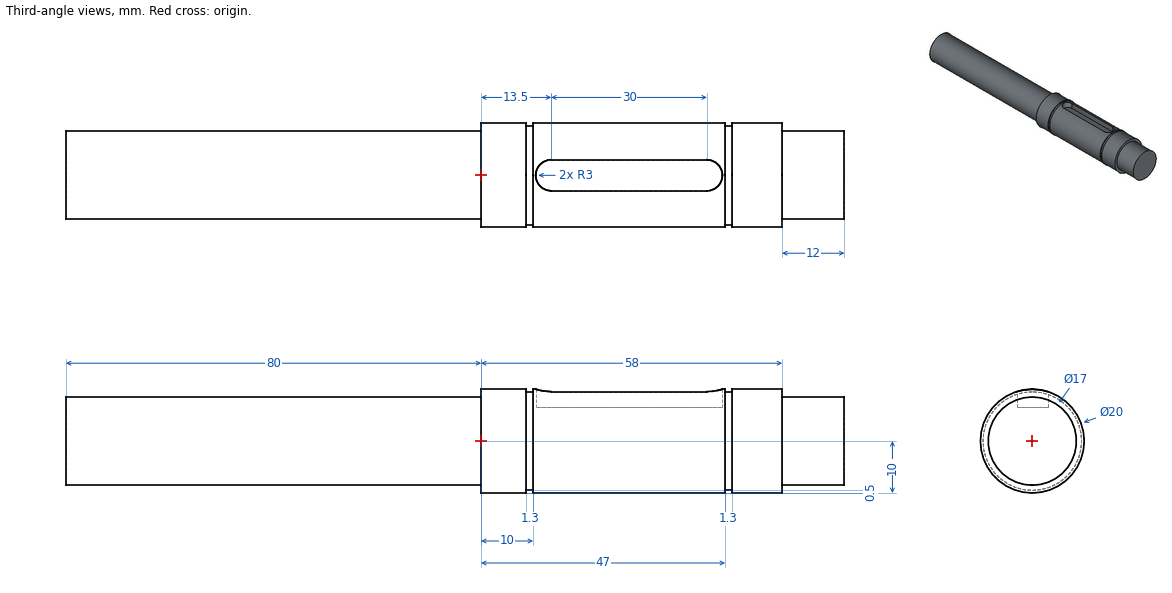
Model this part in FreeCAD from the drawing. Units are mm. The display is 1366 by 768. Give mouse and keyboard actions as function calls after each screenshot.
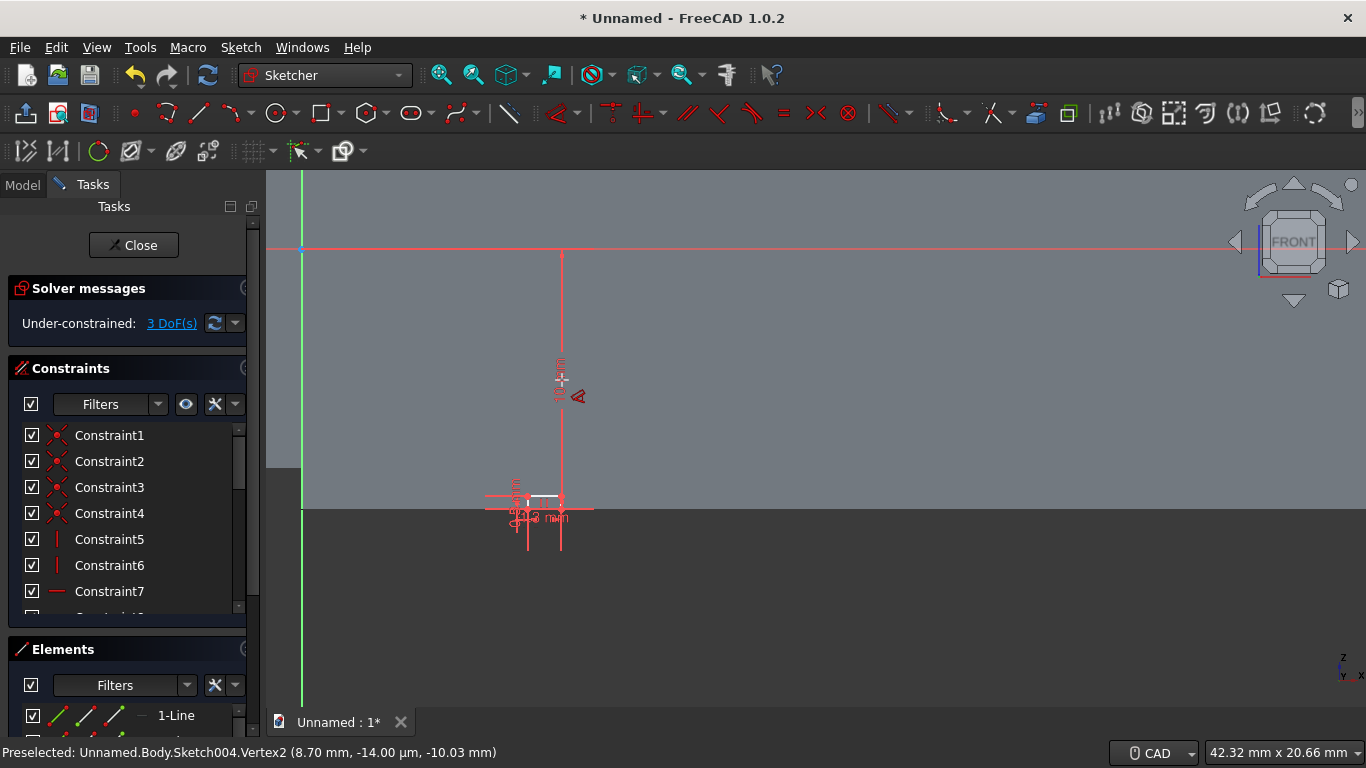
click(561, 509)
click(431, 215)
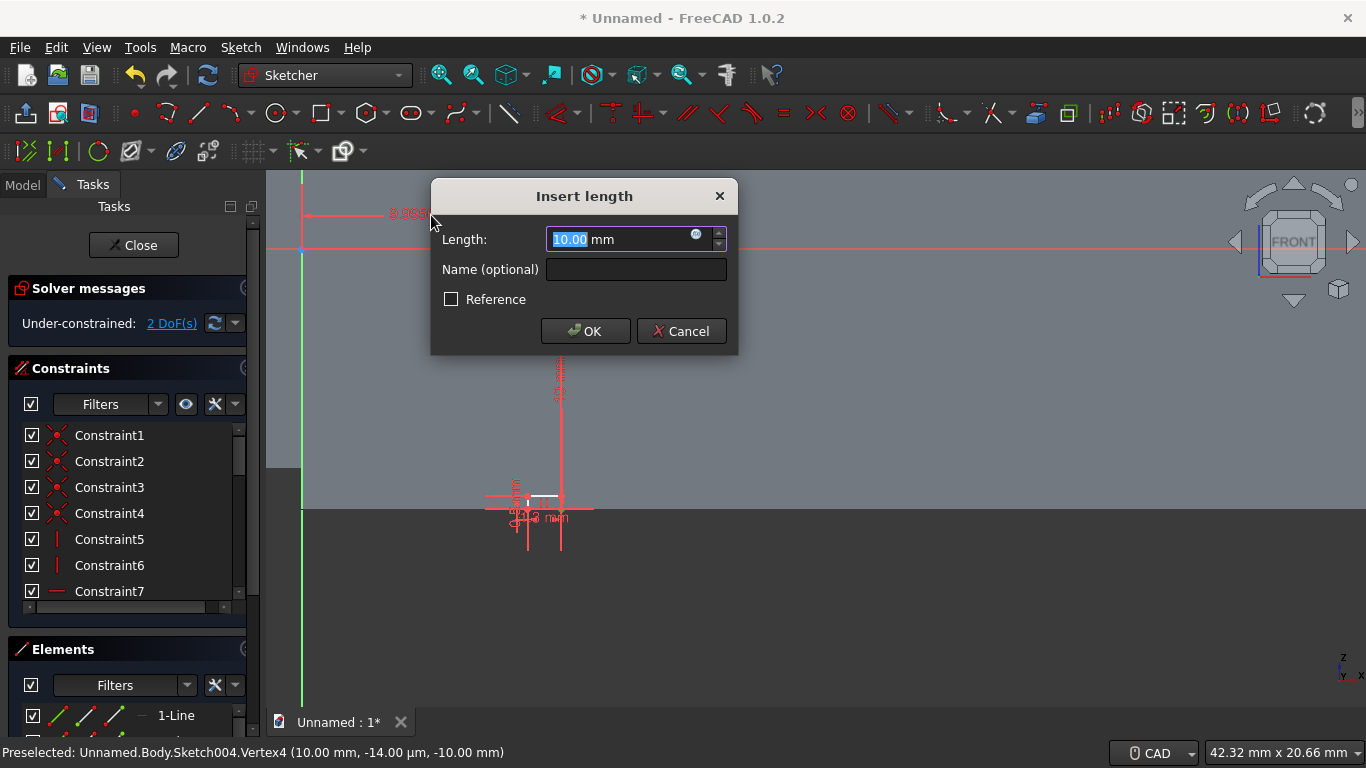
text(10)
key(Return)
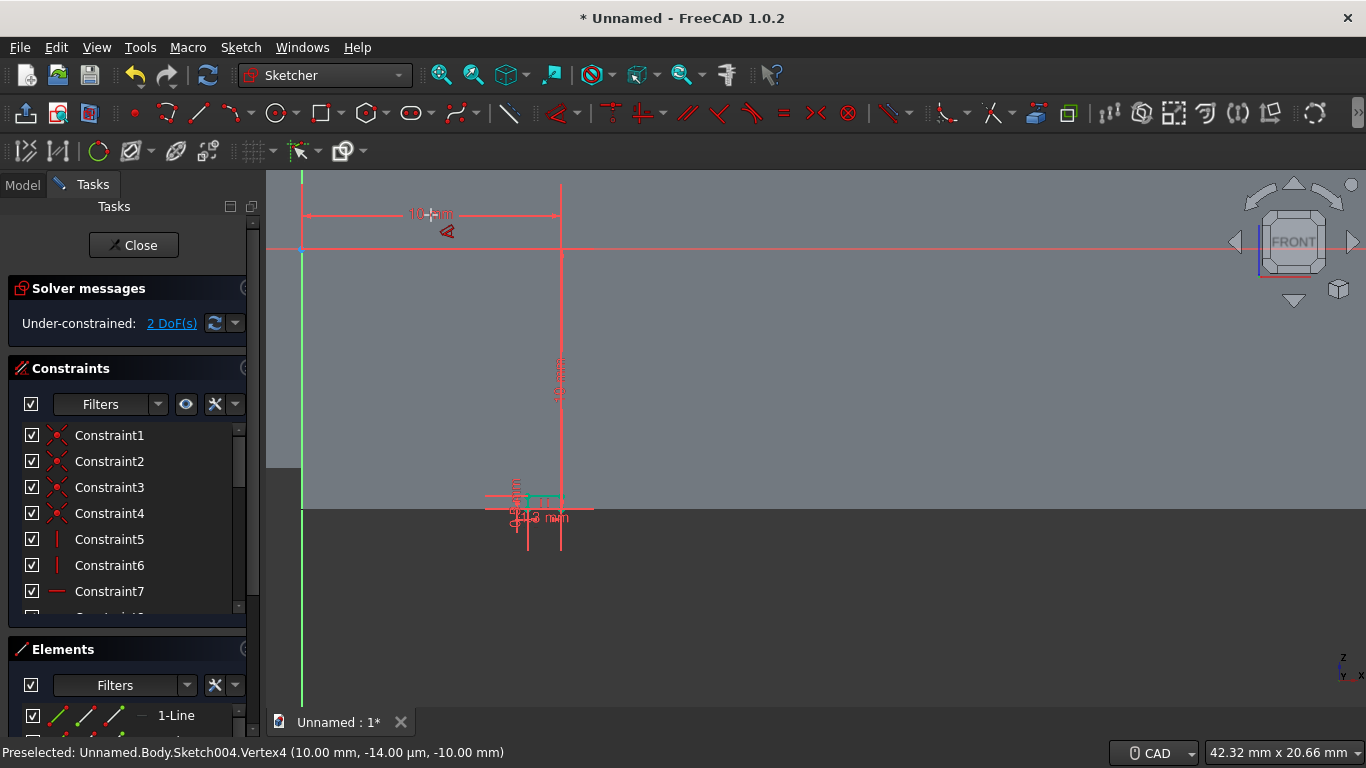
scroll(526, 511, down, 3)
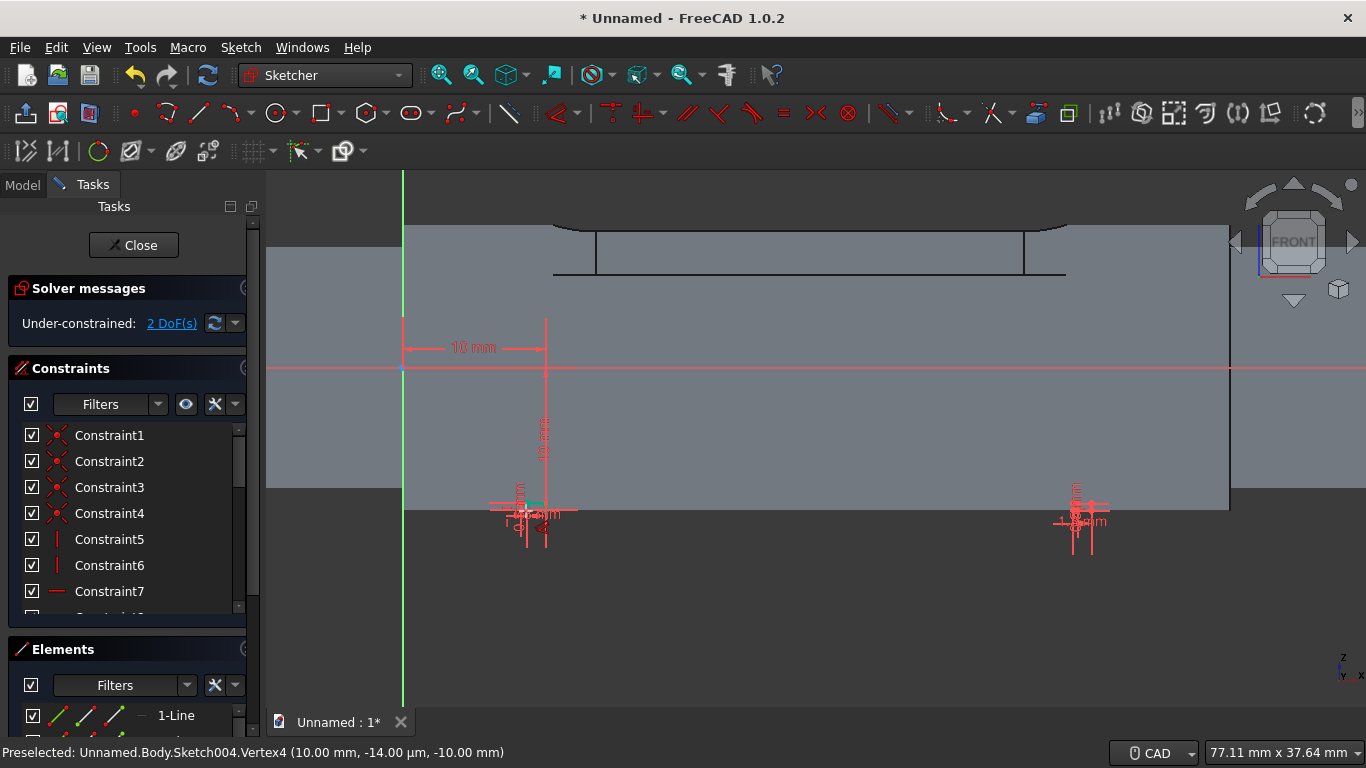
scroll(1073, 504, up, 3)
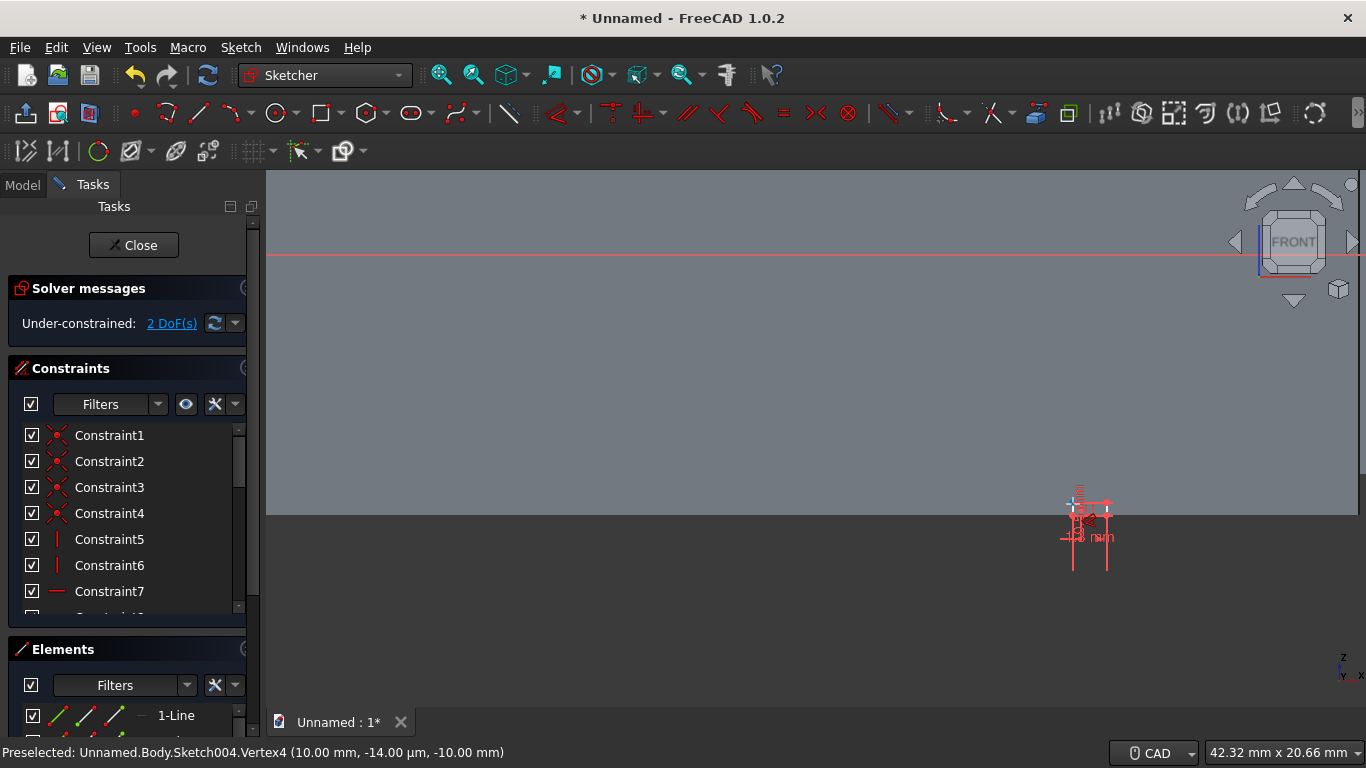
click(1073, 503)
click(683, 221)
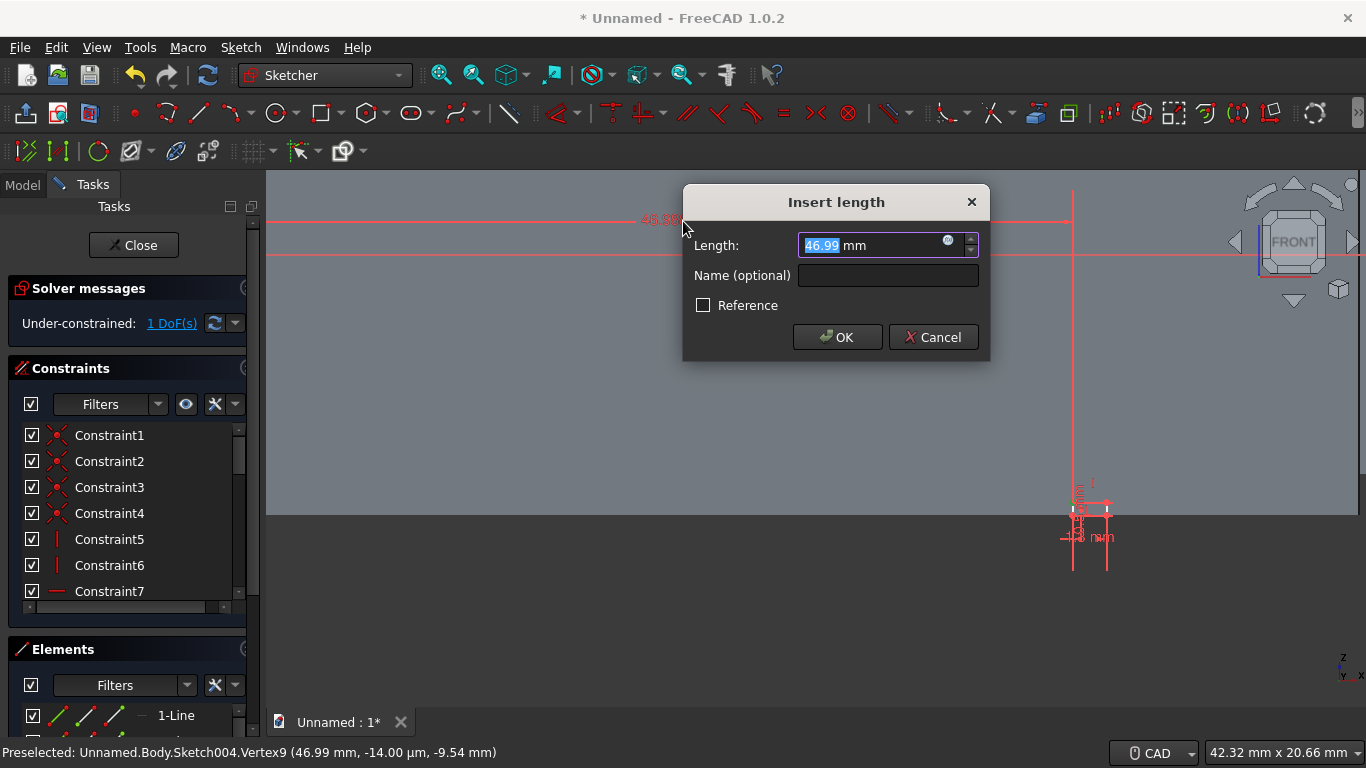
text(47)
key(Return)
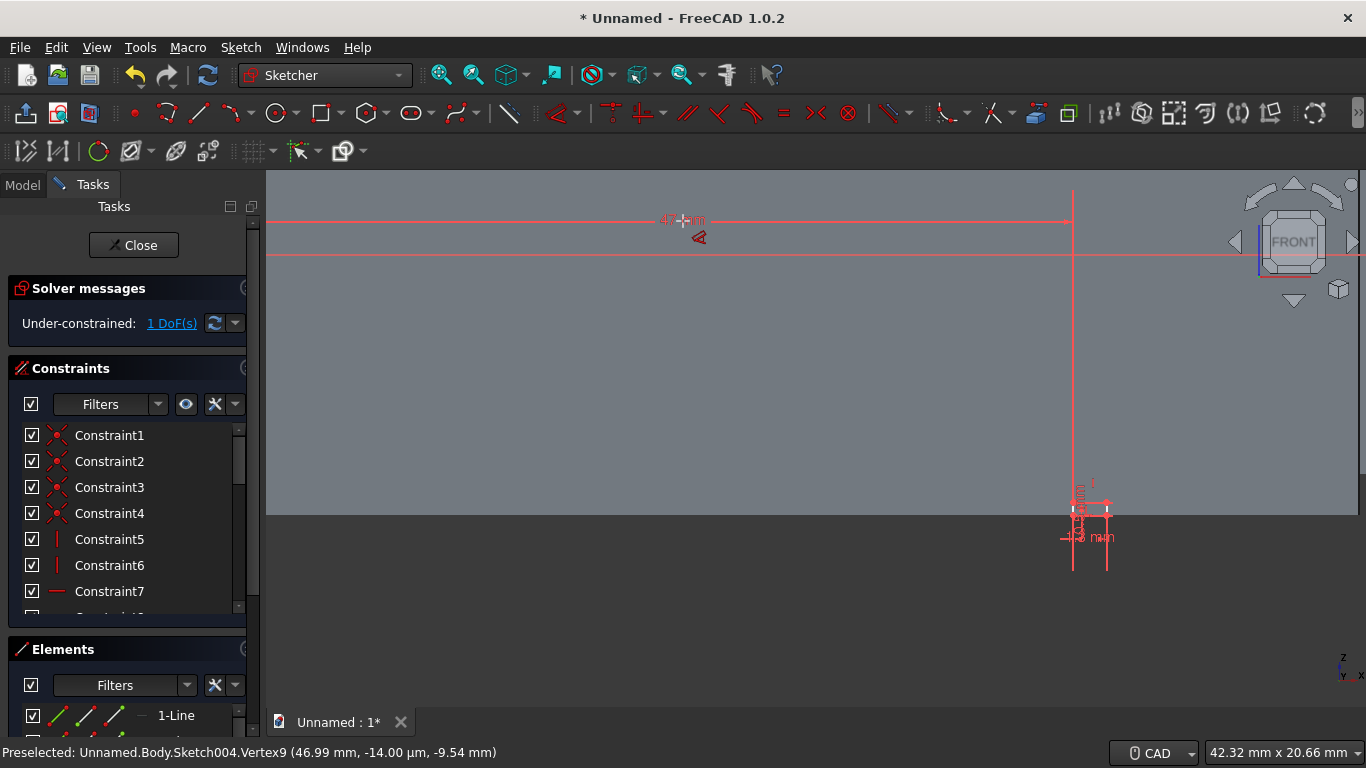
click(1073, 516)
click(1107, 385)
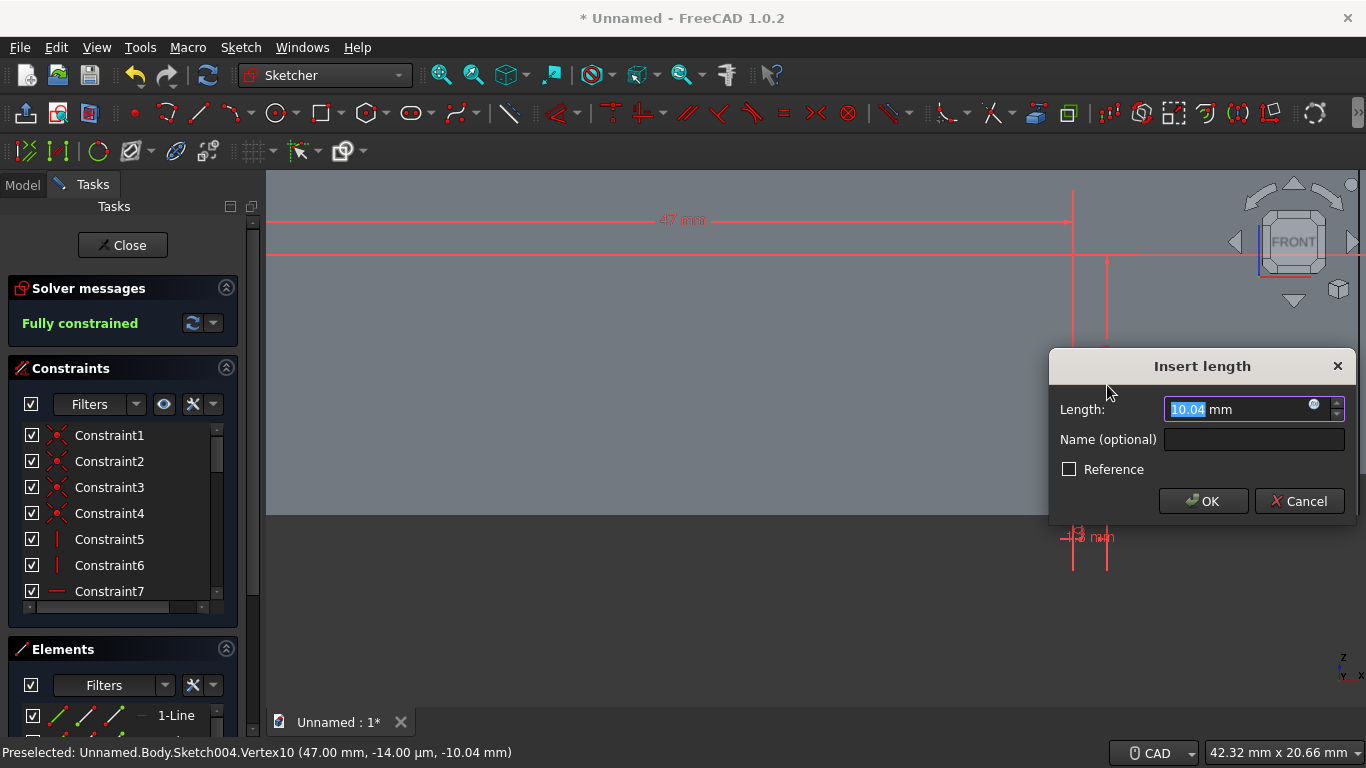
text(10)
key(Return)
key(Escape)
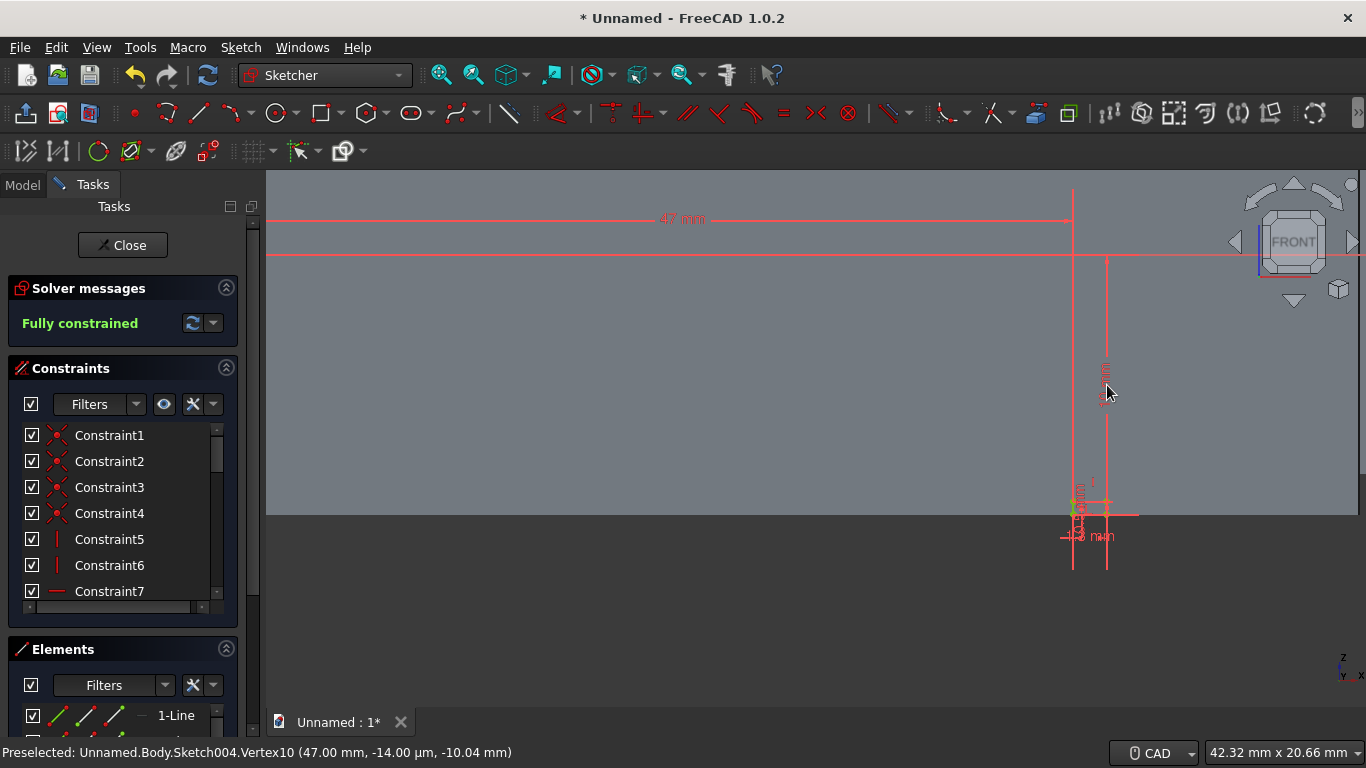
click(123, 245)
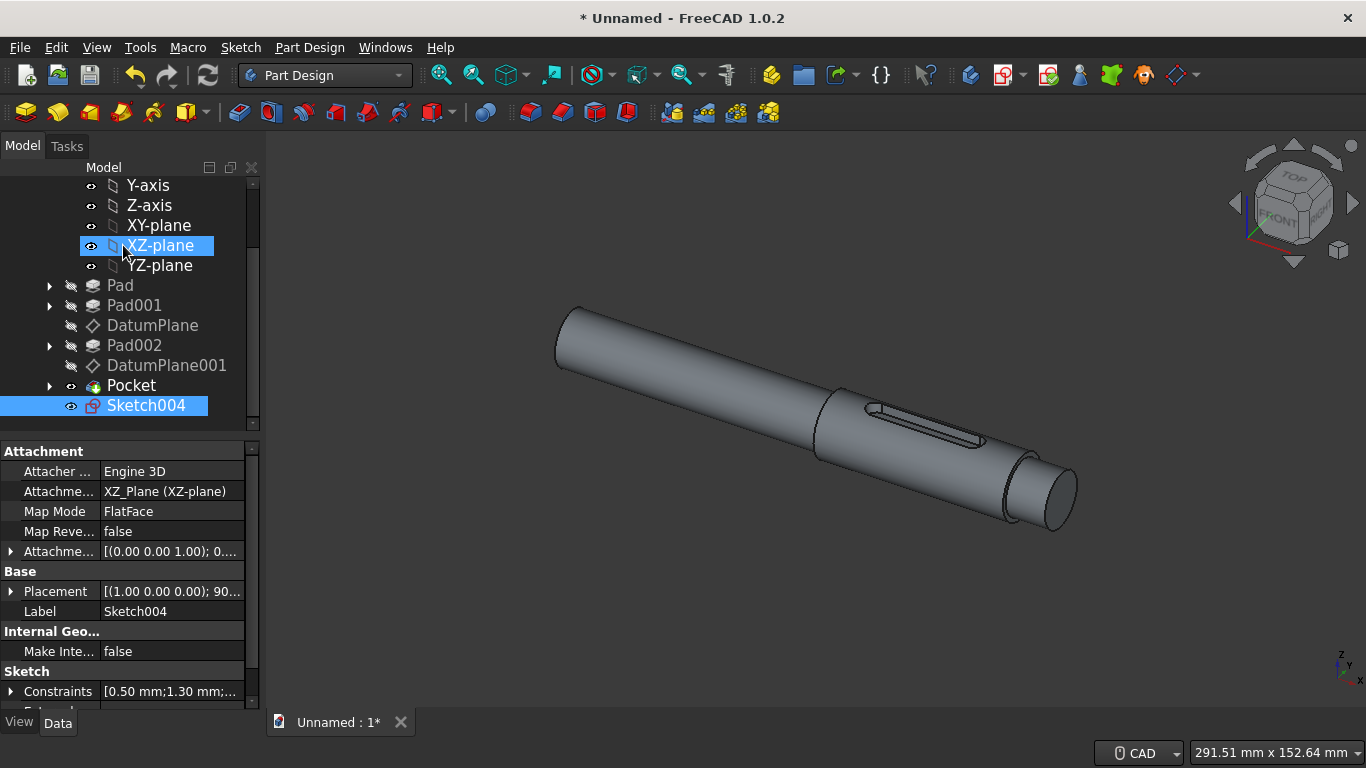
click(304, 112)